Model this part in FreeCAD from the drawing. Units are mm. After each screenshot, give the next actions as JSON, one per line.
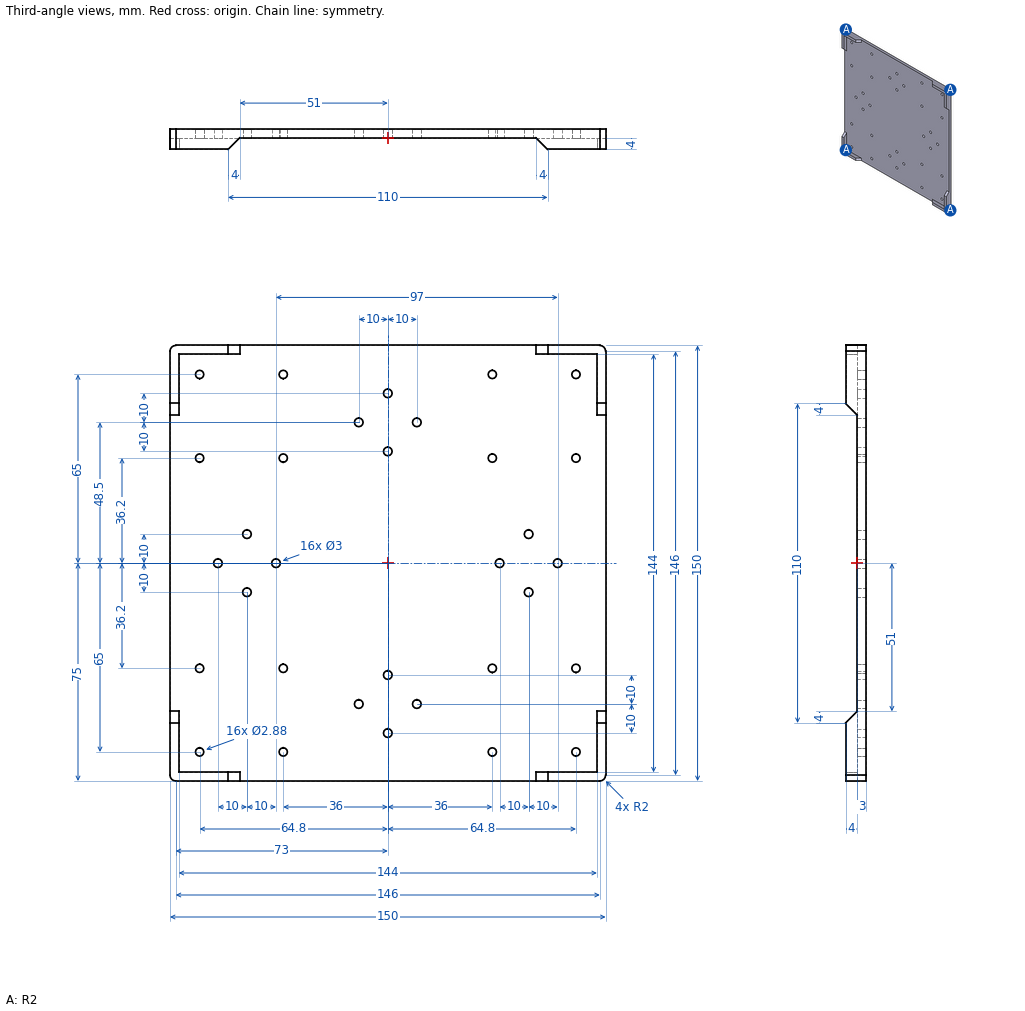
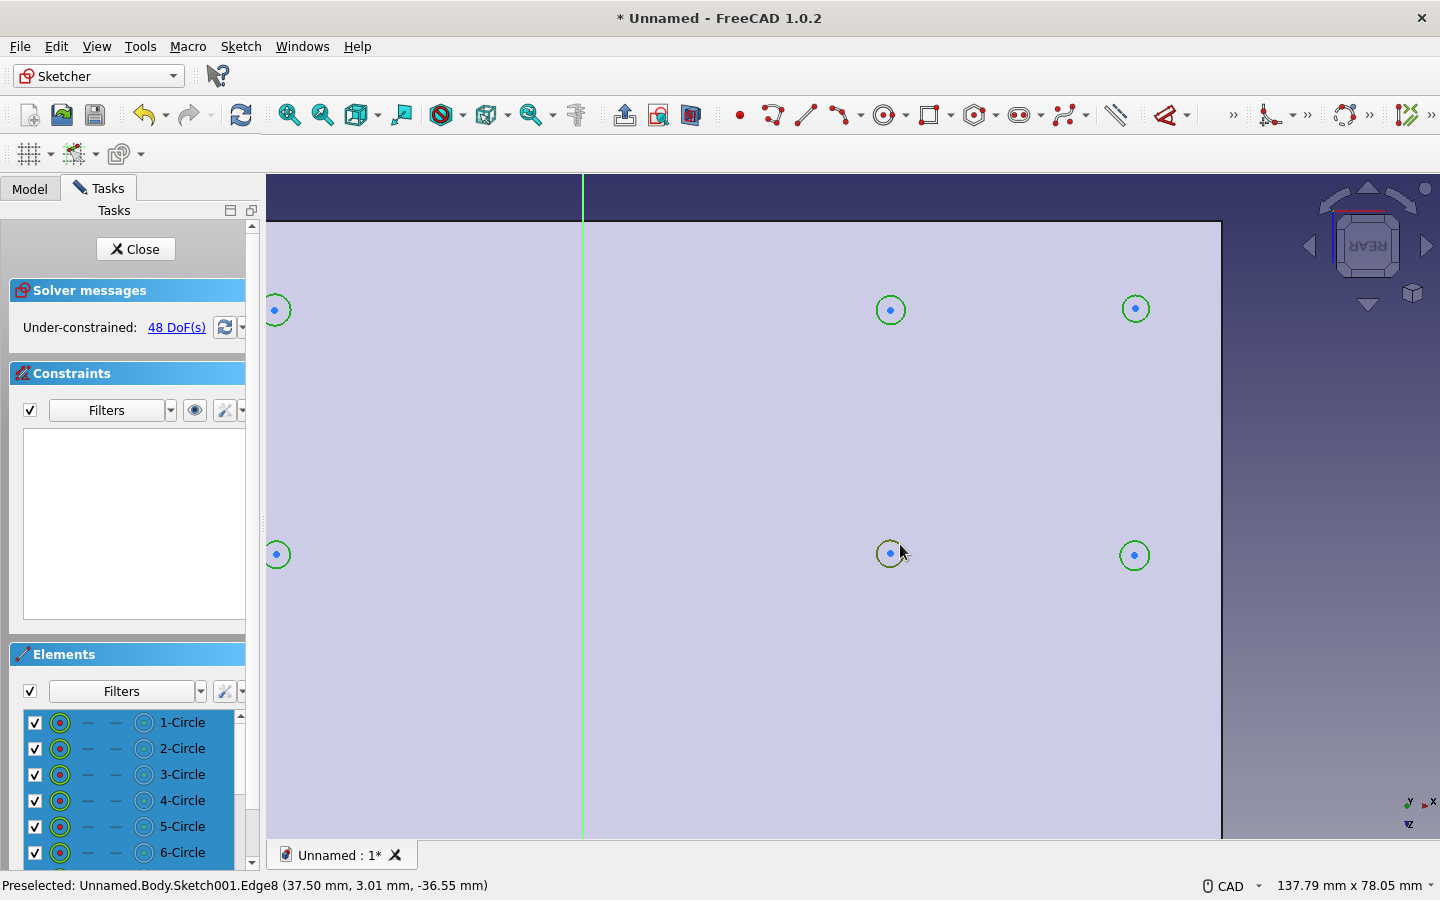
{"action": "scroll", "coordinate": [902, 301], "scroll_direction": "down", "scroll_amount": 5}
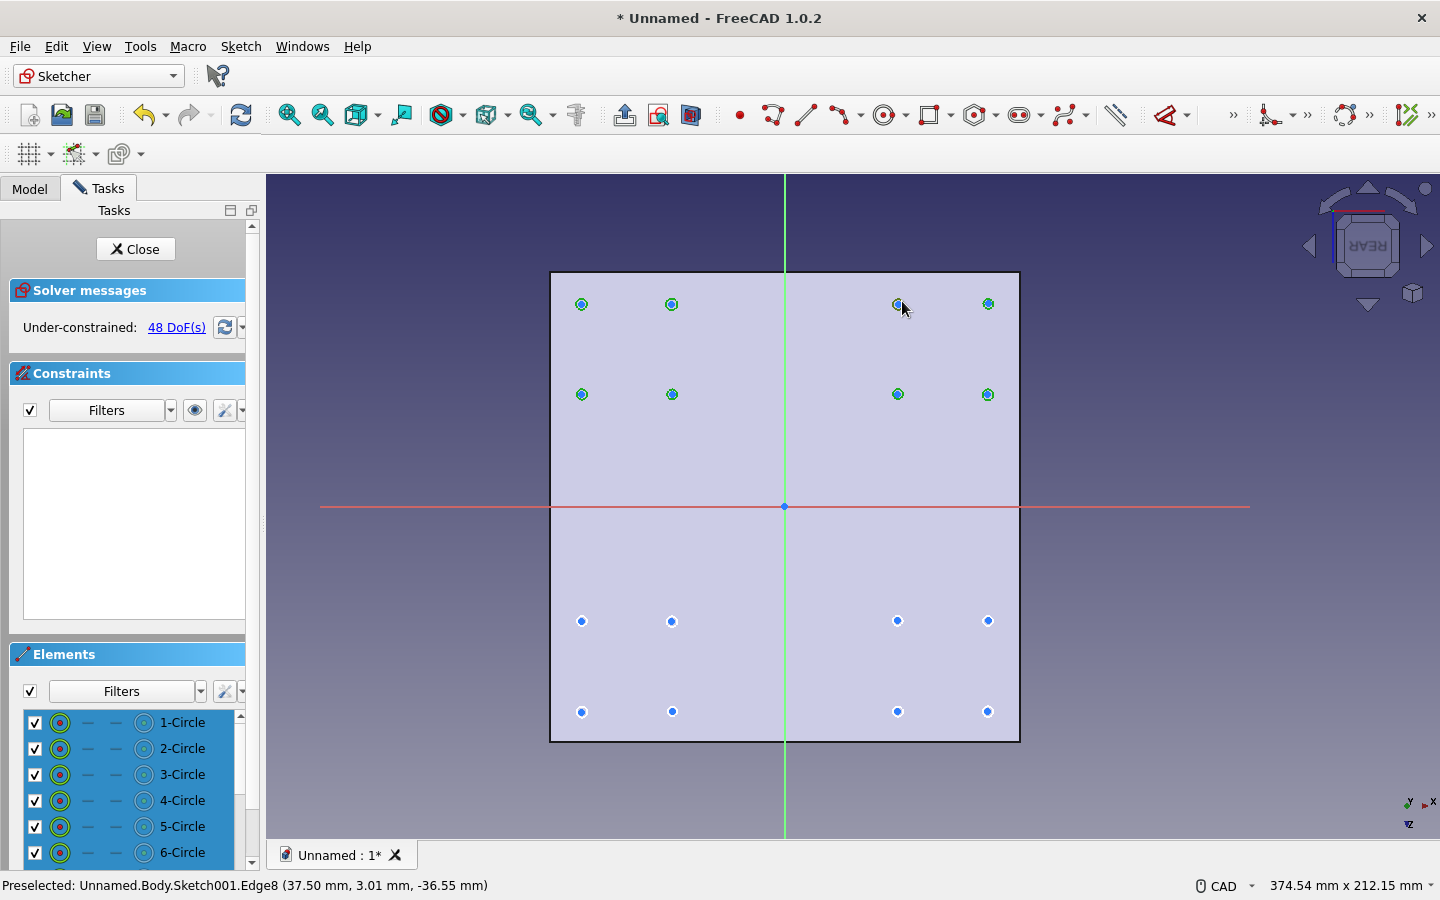
{"action": "scroll", "coordinate": [585, 618], "scroll_direction": "up", "scroll_amount": 6}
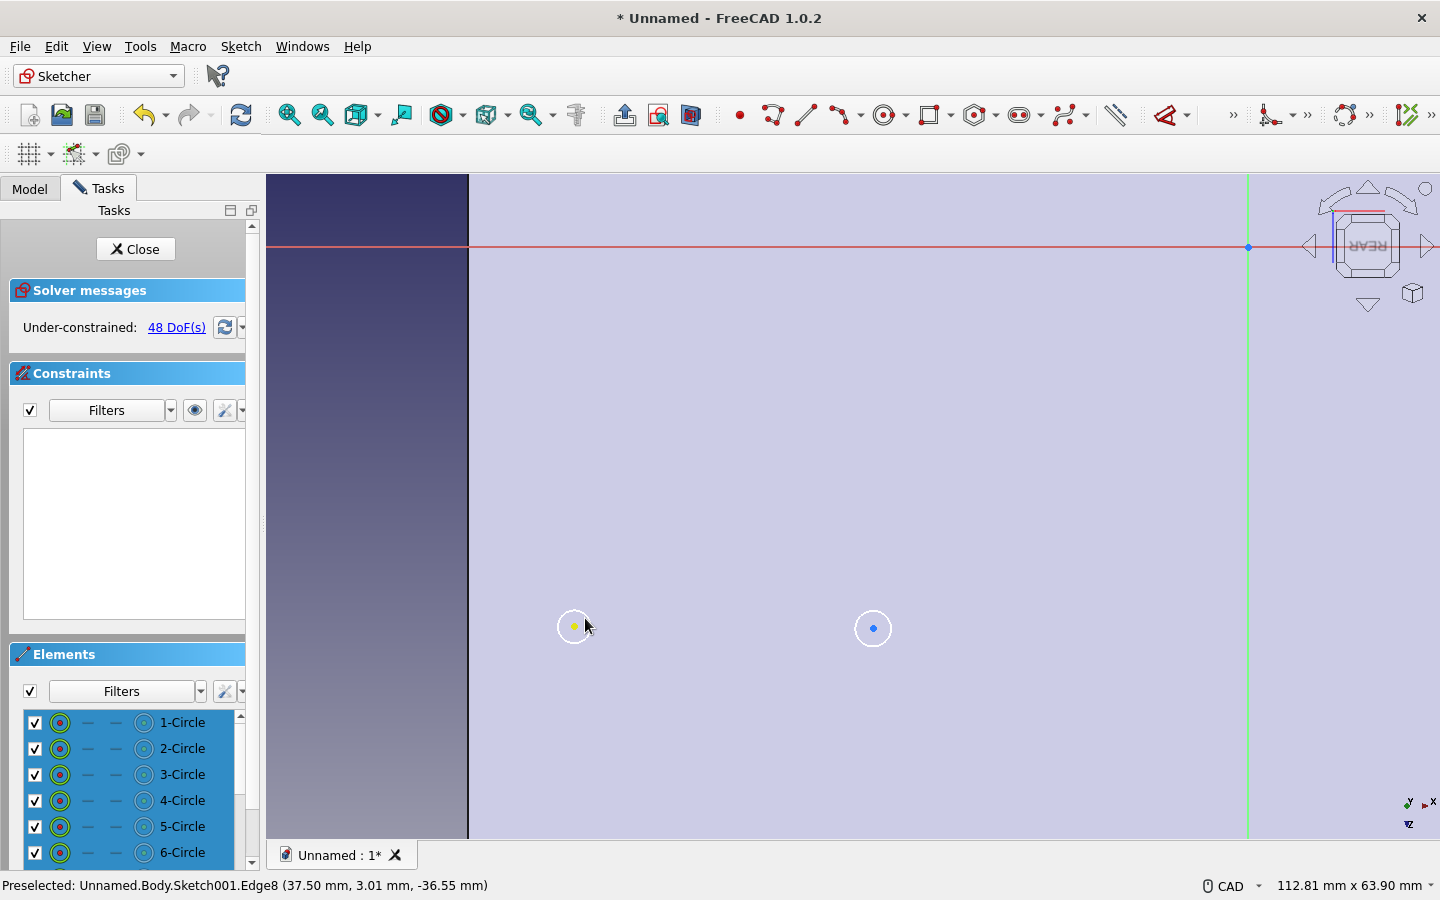
{"action": "left_click", "coordinate": [586, 615]}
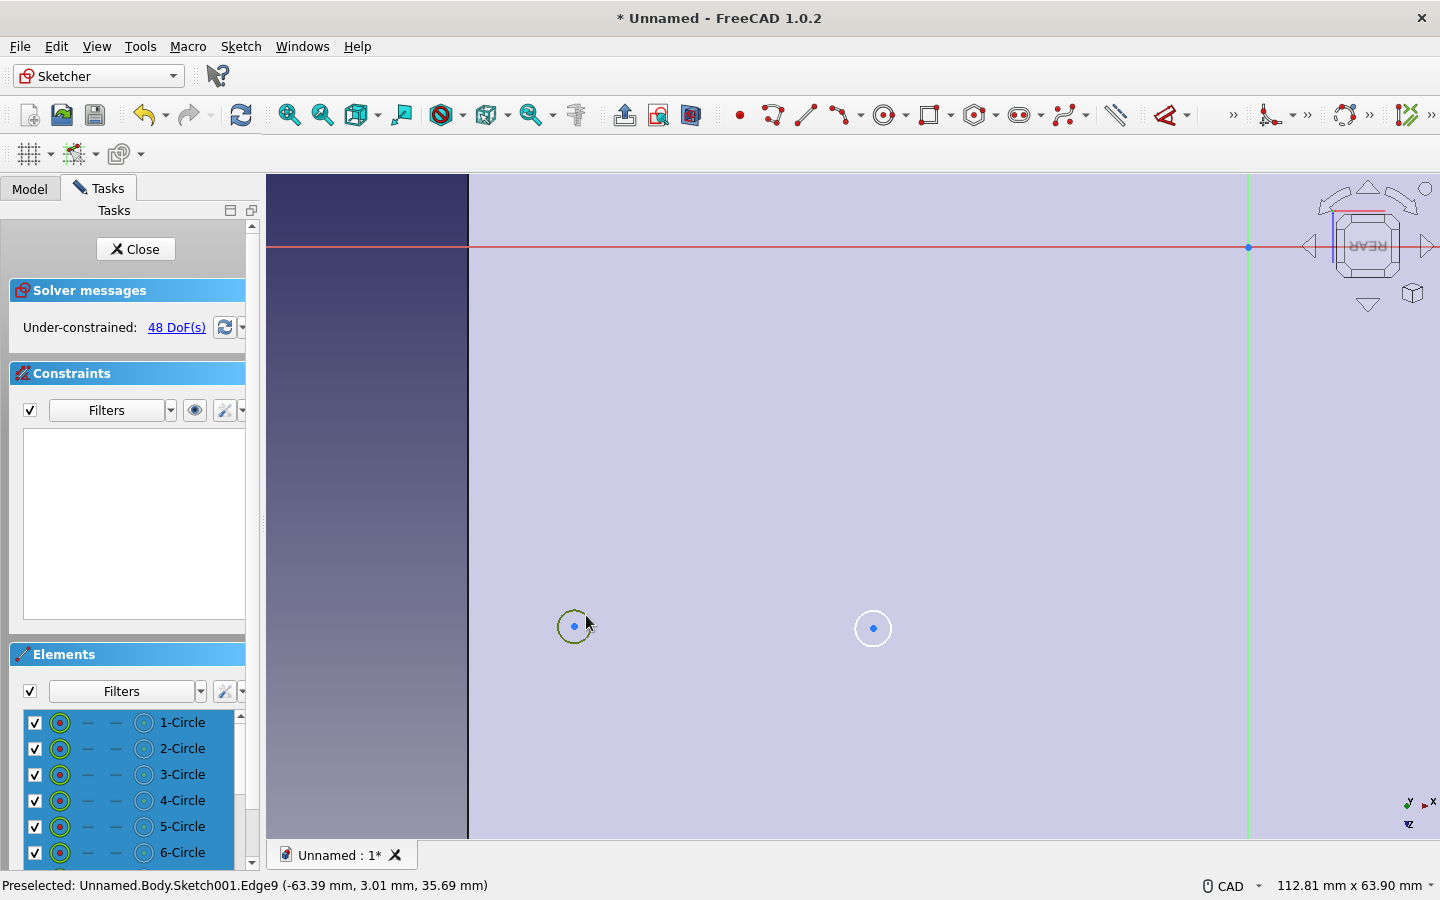
{"action": "scroll", "coordinate": [585, 618], "scroll_direction": "down", "scroll_amount": 6}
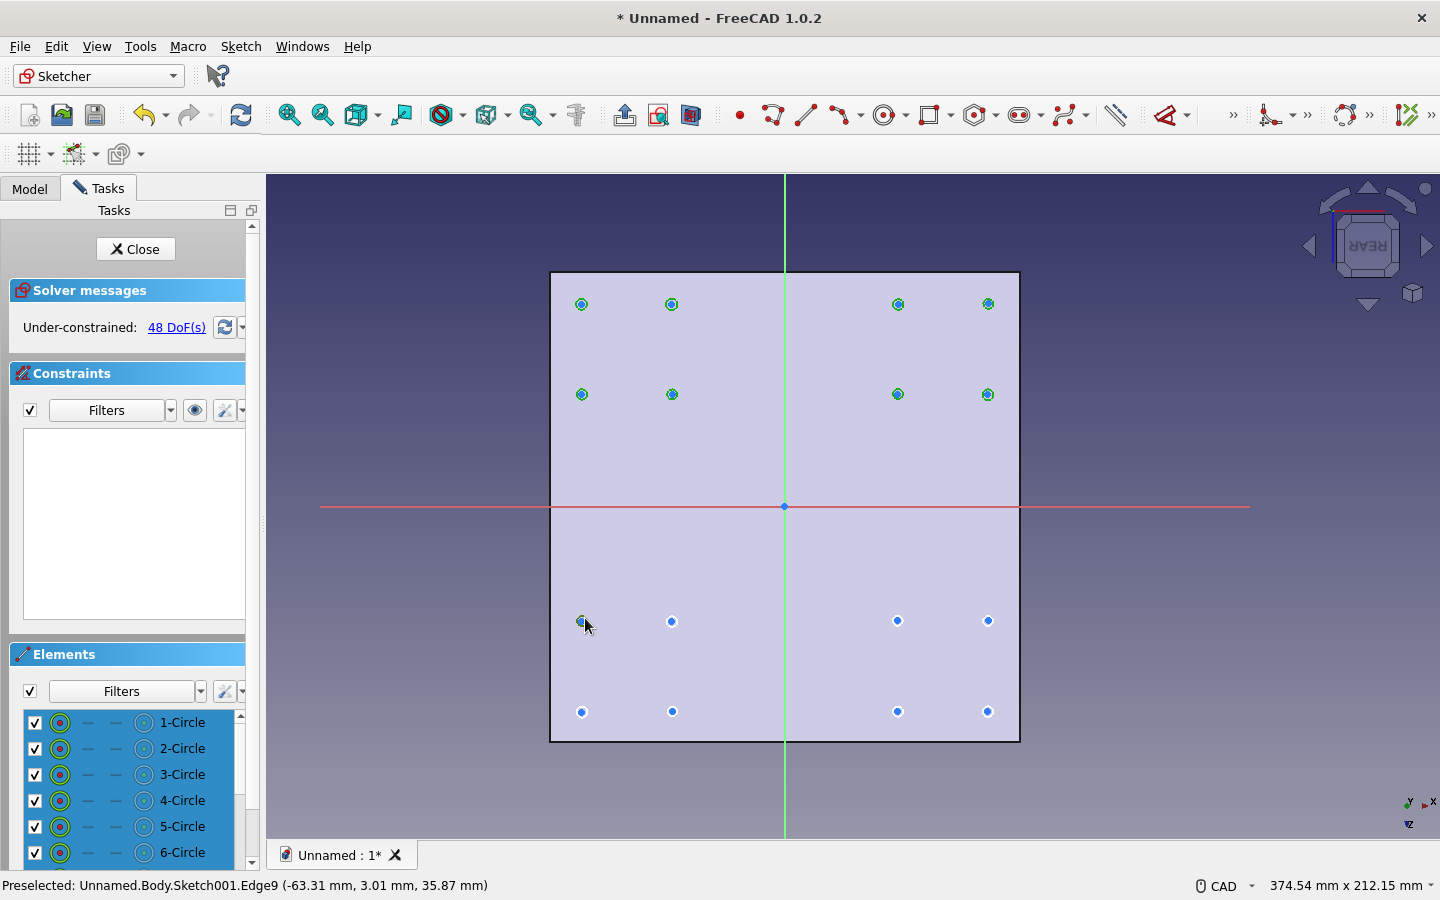
{"action": "scroll", "coordinate": [586, 708], "scroll_direction": "up", "scroll_amount": 5}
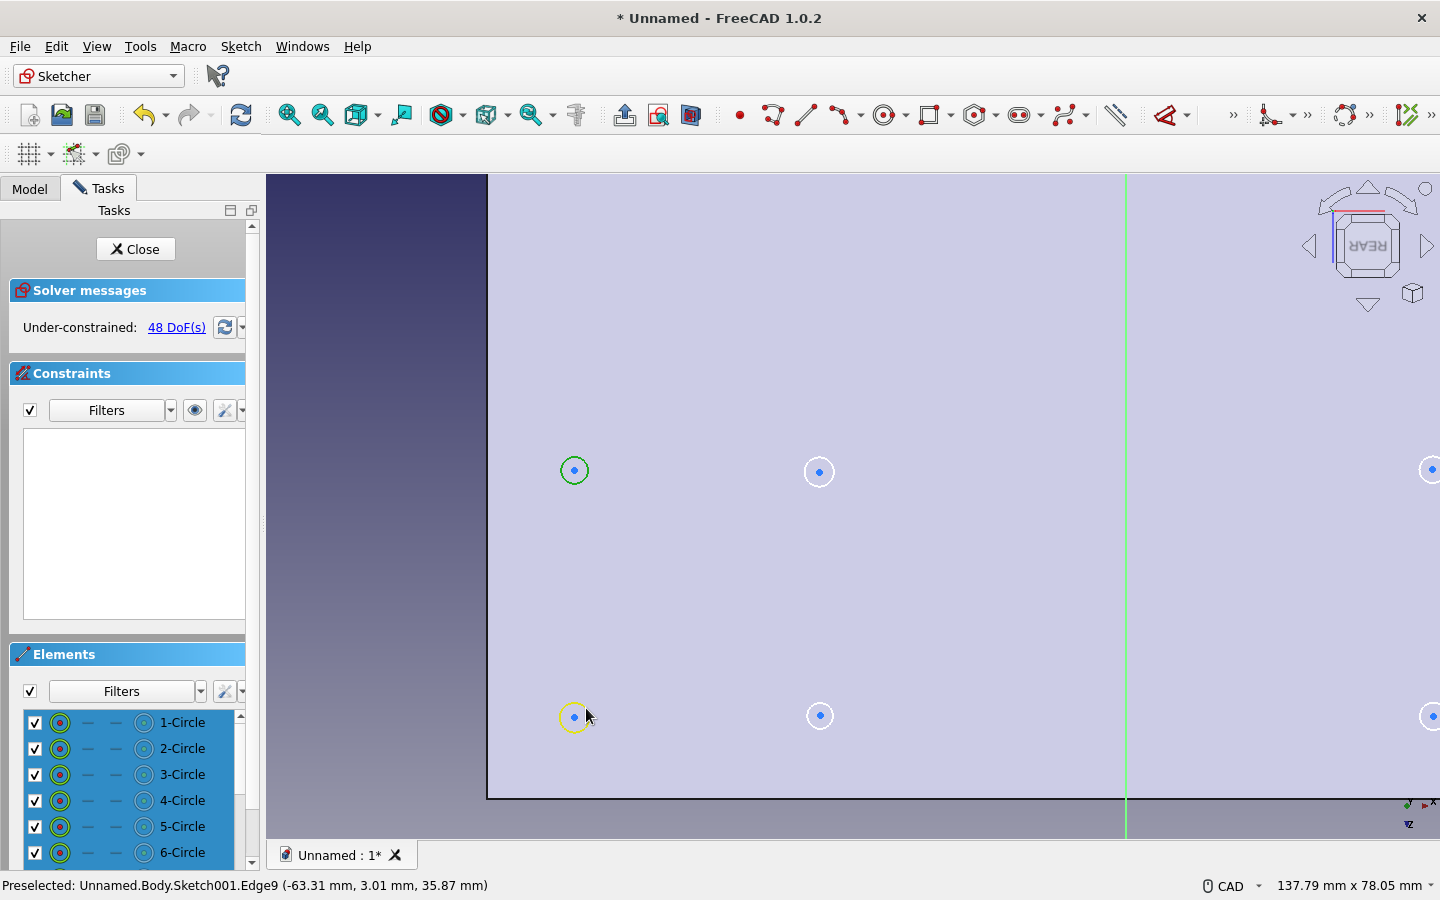
{"action": "left_click", "coordinate": [585, 707]}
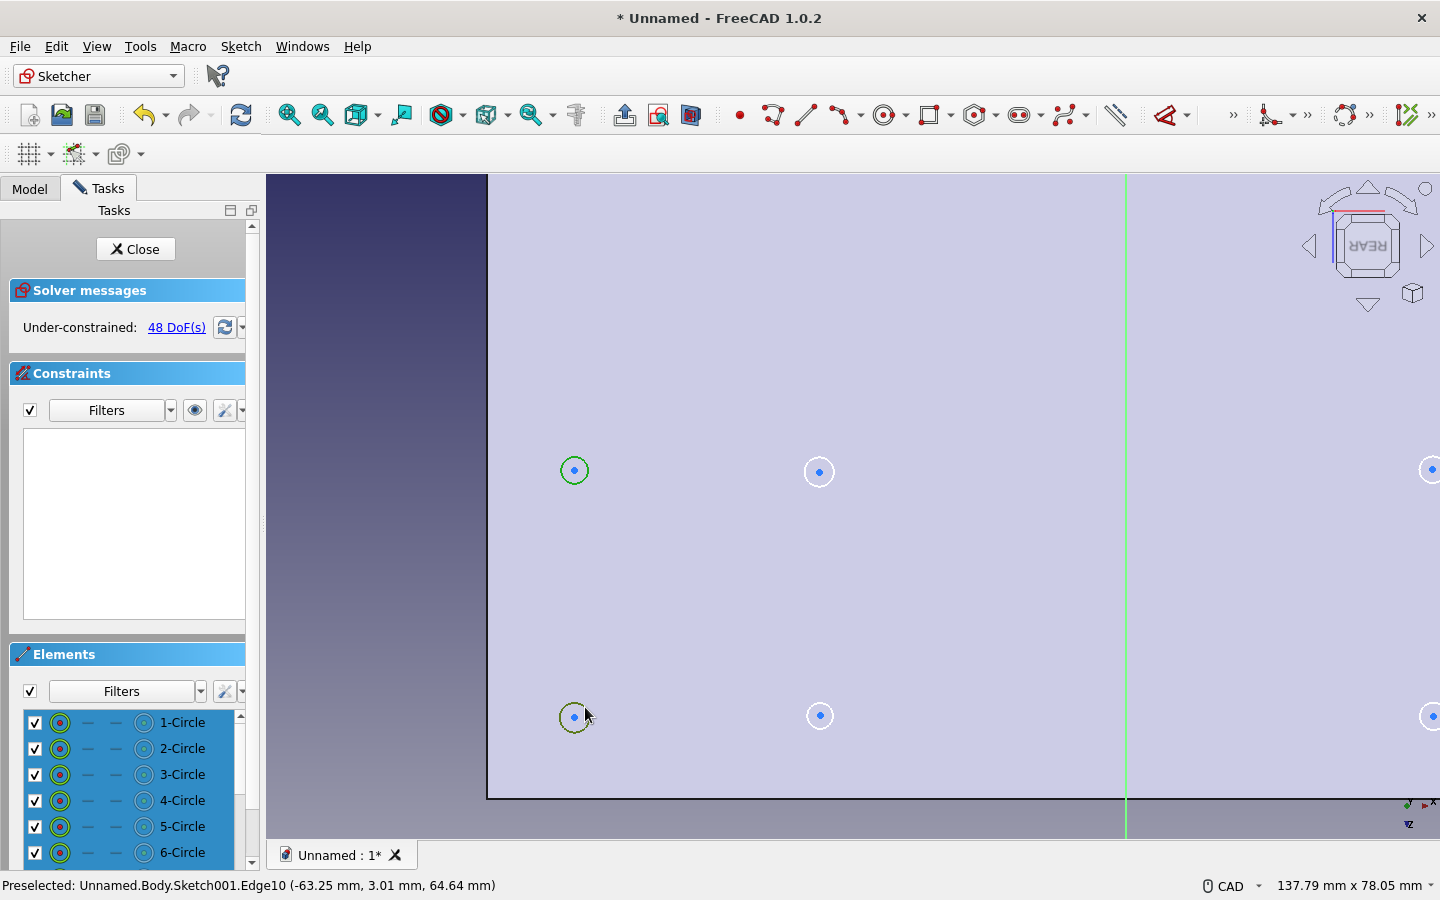
{"action": "left_click", "coordinate": [829, 707]}